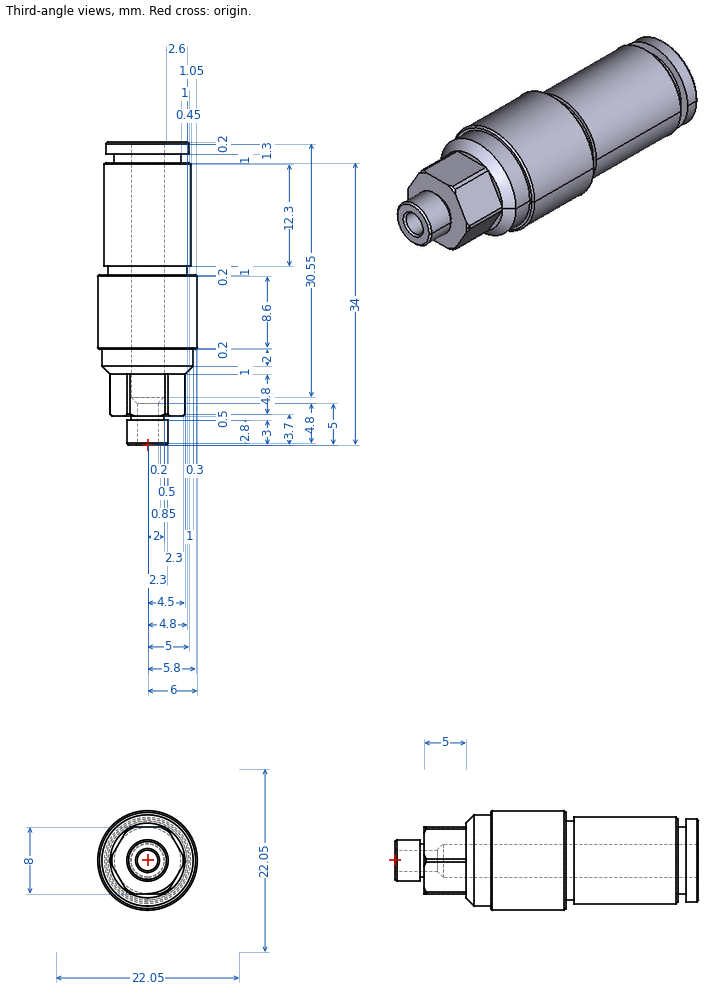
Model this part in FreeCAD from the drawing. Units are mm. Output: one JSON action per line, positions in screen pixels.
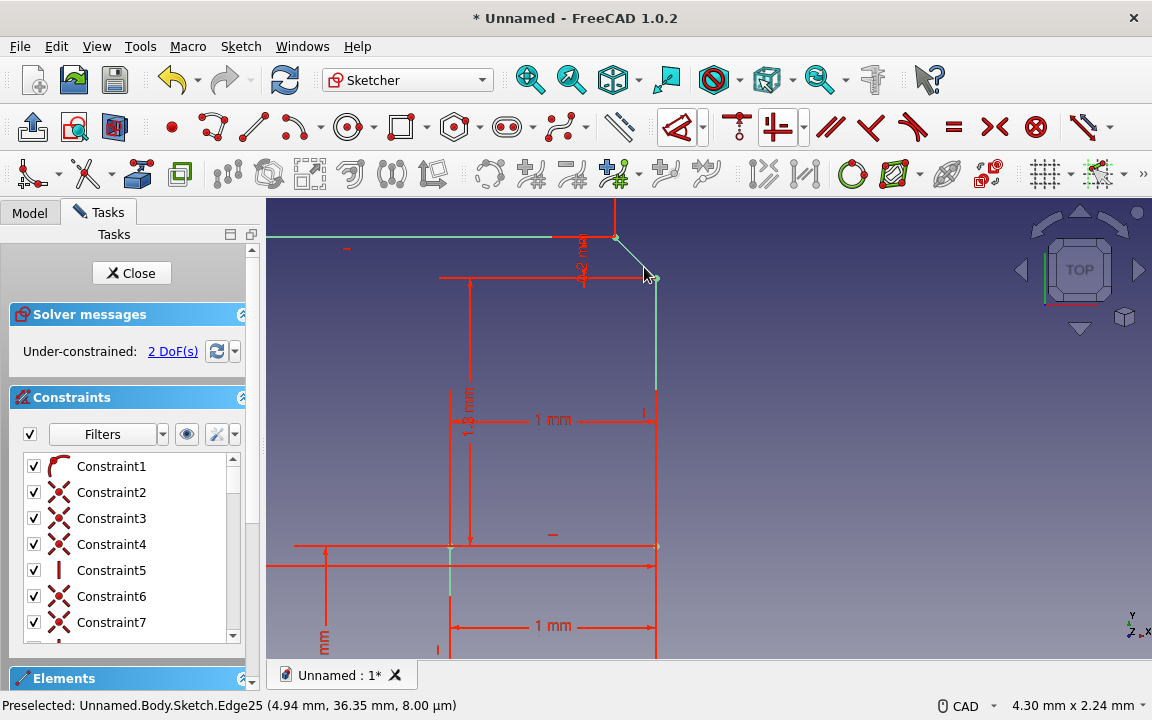
{"action": "scroll", "coordinate": [657, 277], "scroll_direction": "down", "scroll_amount": 16}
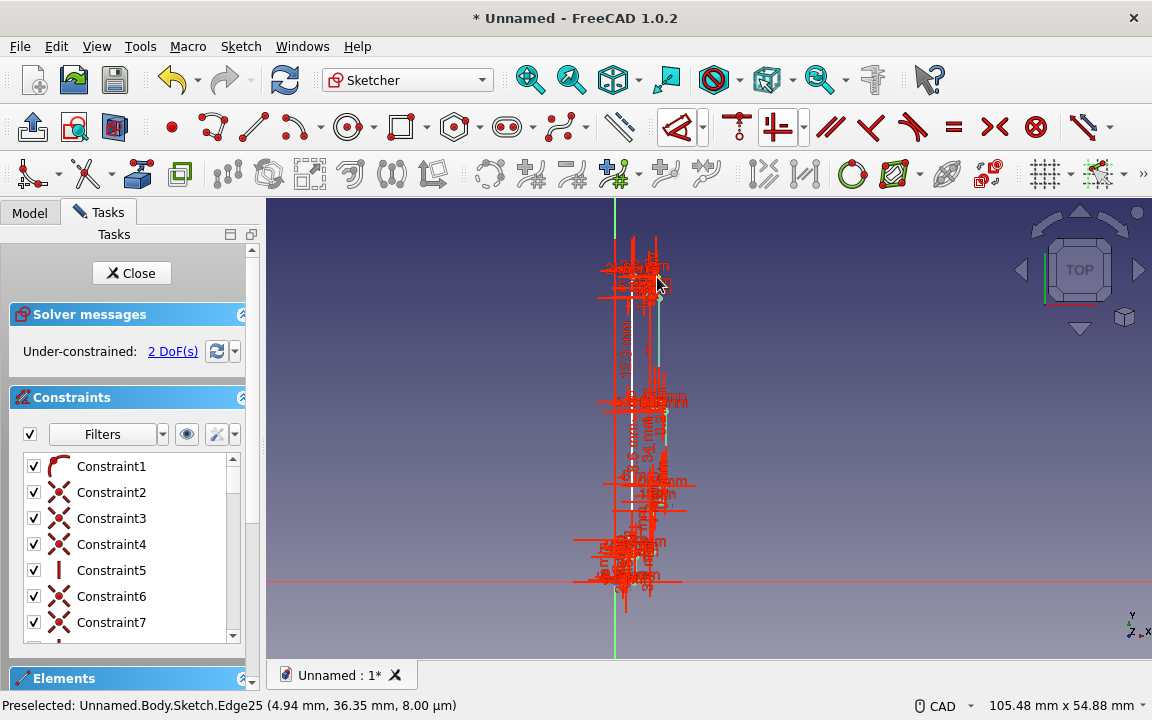
{"action": "scroll", "coordinate": [633, 276], "scroll_direction": "up", "scroll_amount": 16}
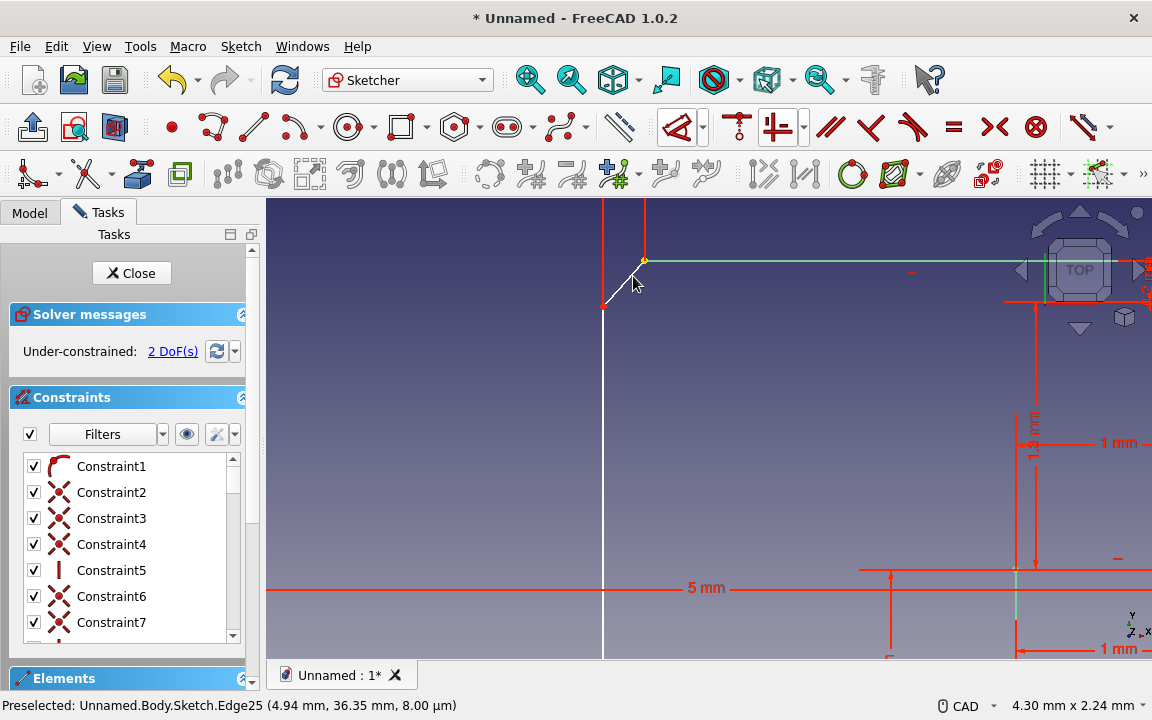
{"action": "left_click", "coordinate": [632, 274]}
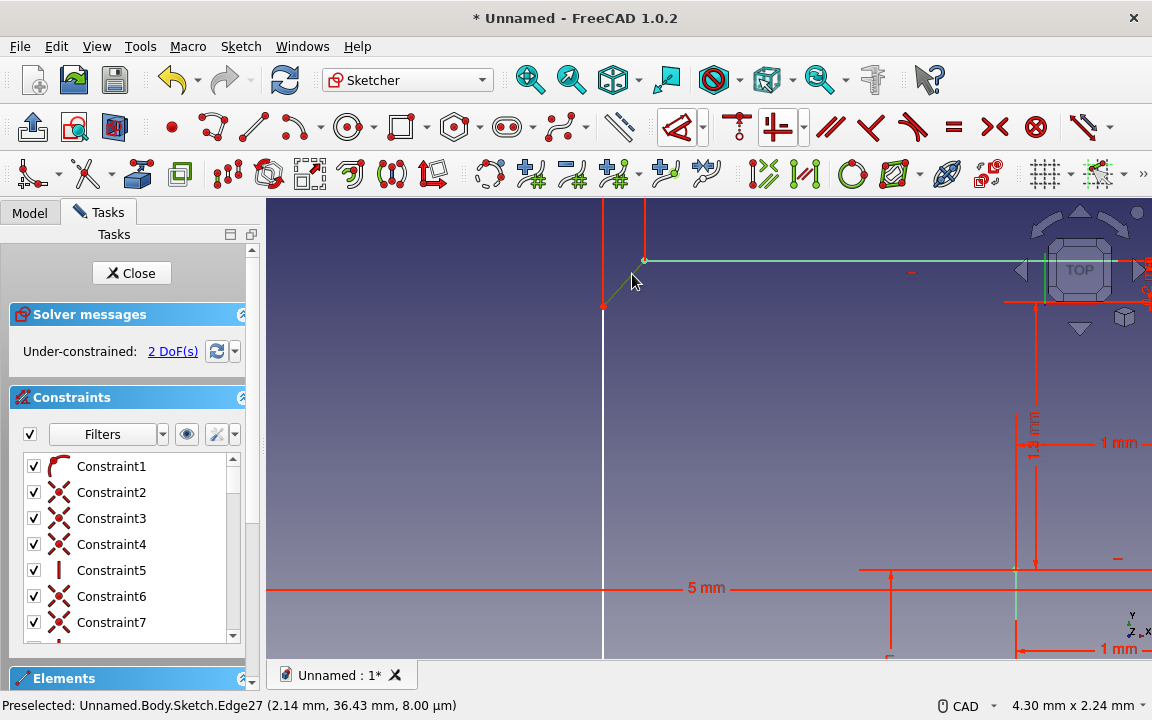
{"action": "left_click", "coordinate": [702, 128]}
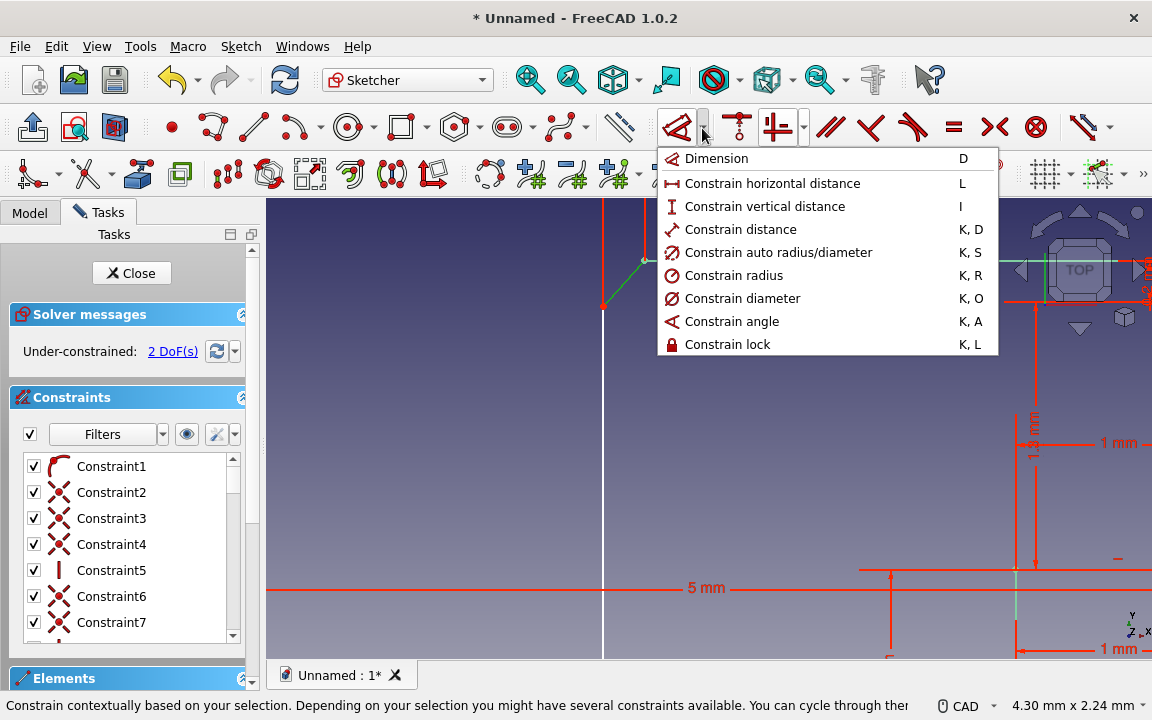
{"action": "left_click", "coordinate": [828, 206]}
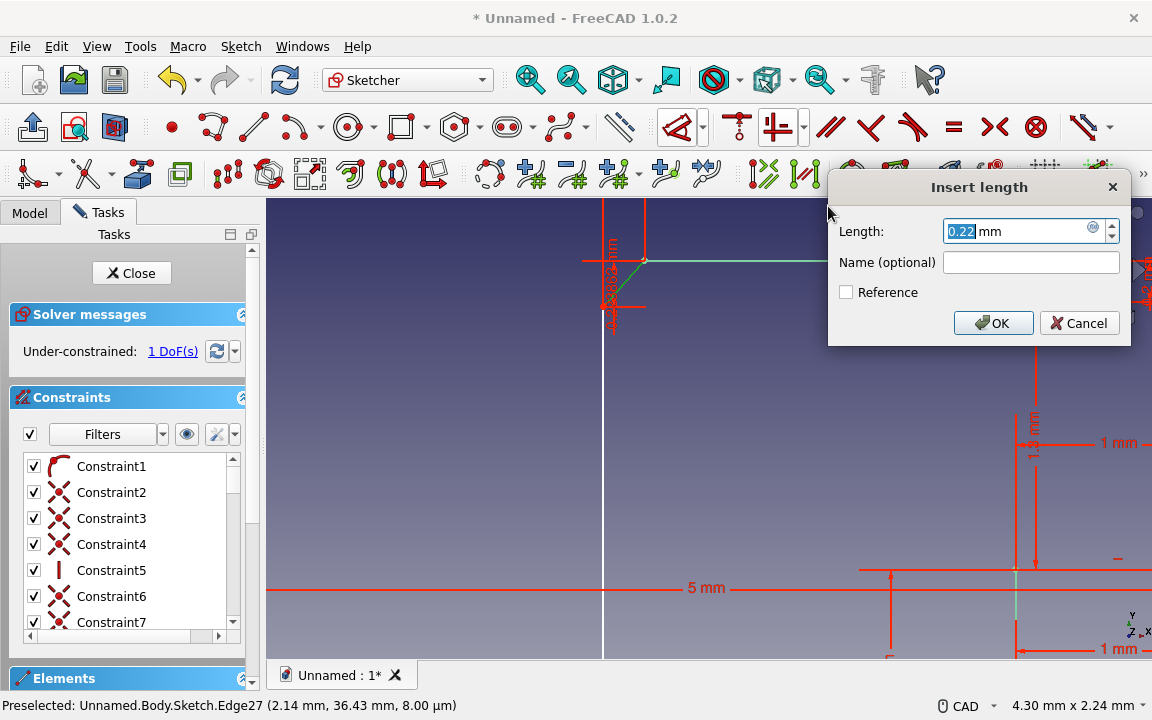
{"action": "type", "text": "0.2"}
{"action": "key", "text": "Return"}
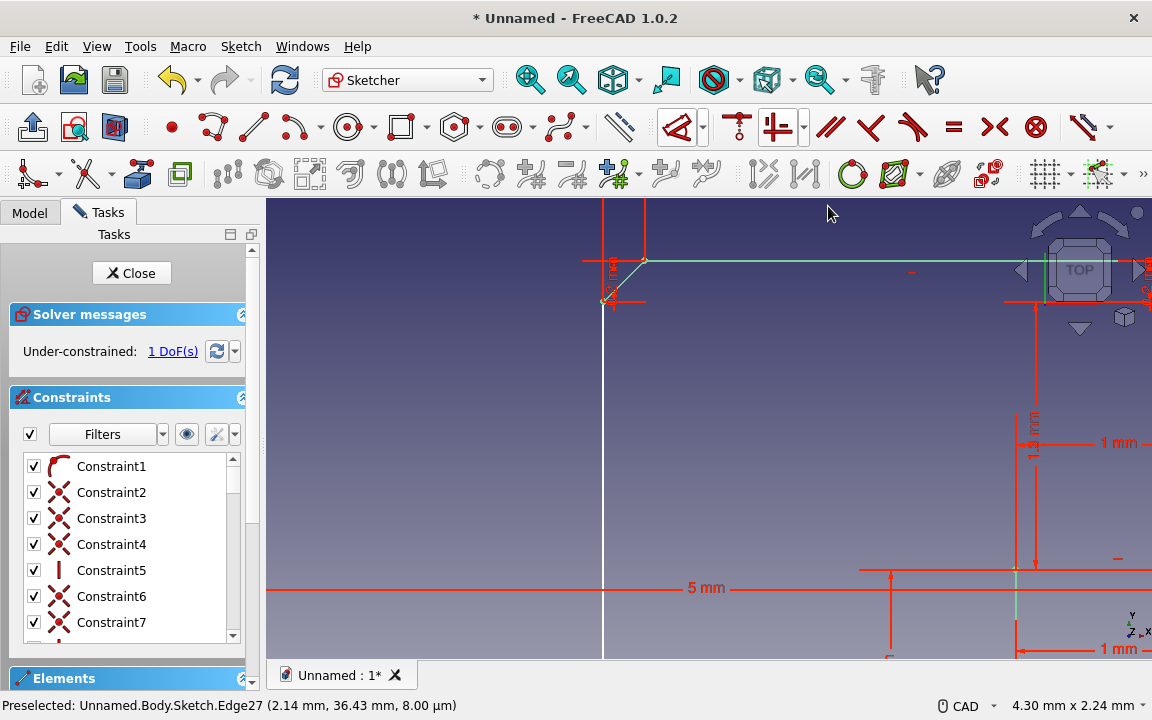
{"action": "scroll", "coordinate": [633, 276], "scroll_direction": "down", "scroll_amount": 16}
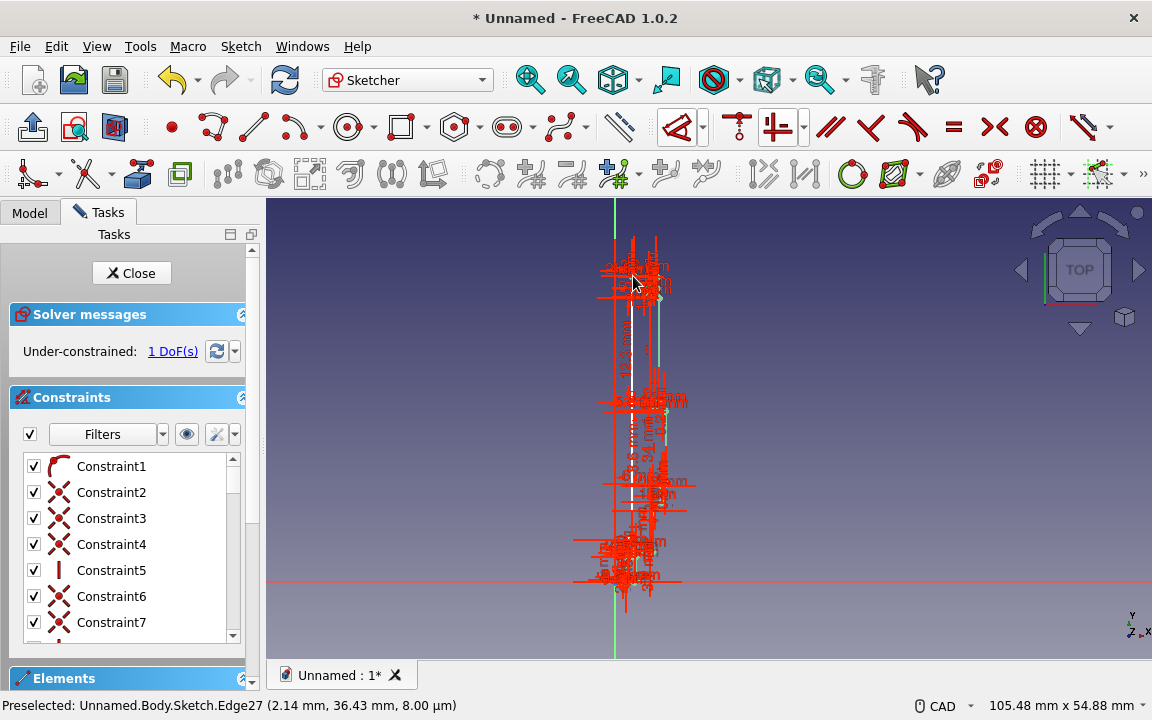
{"action": "left_click", "coordinate": [632, 380]}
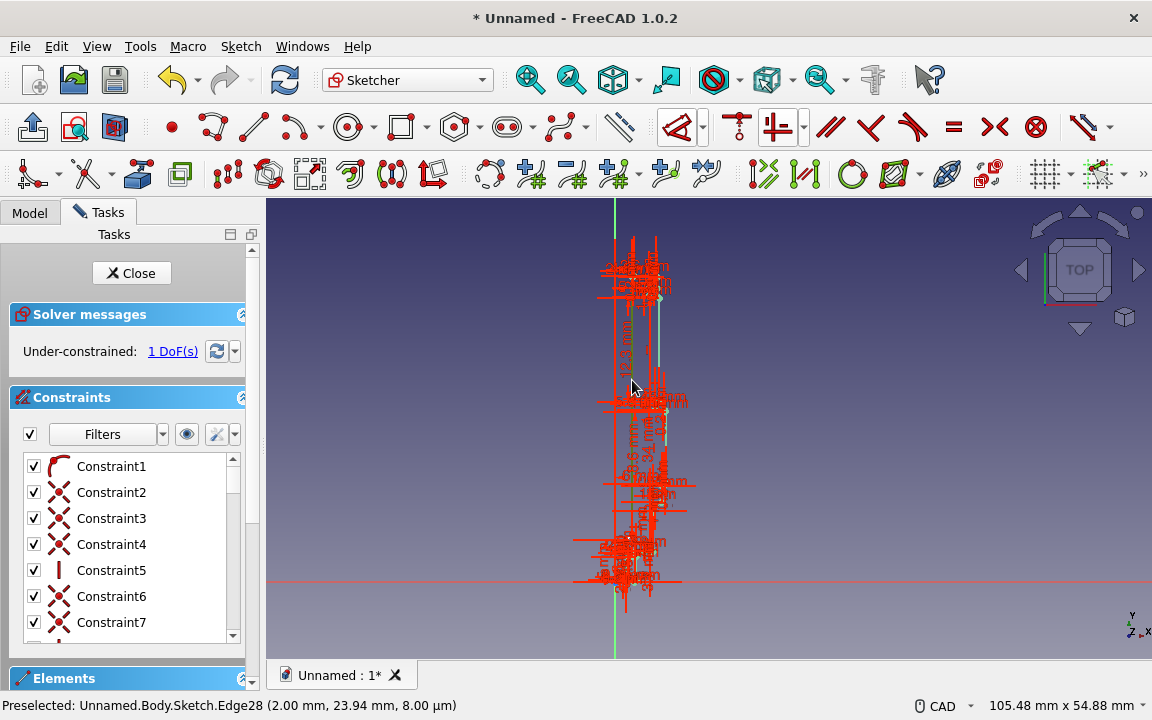
{"action": "key", "text": "i"}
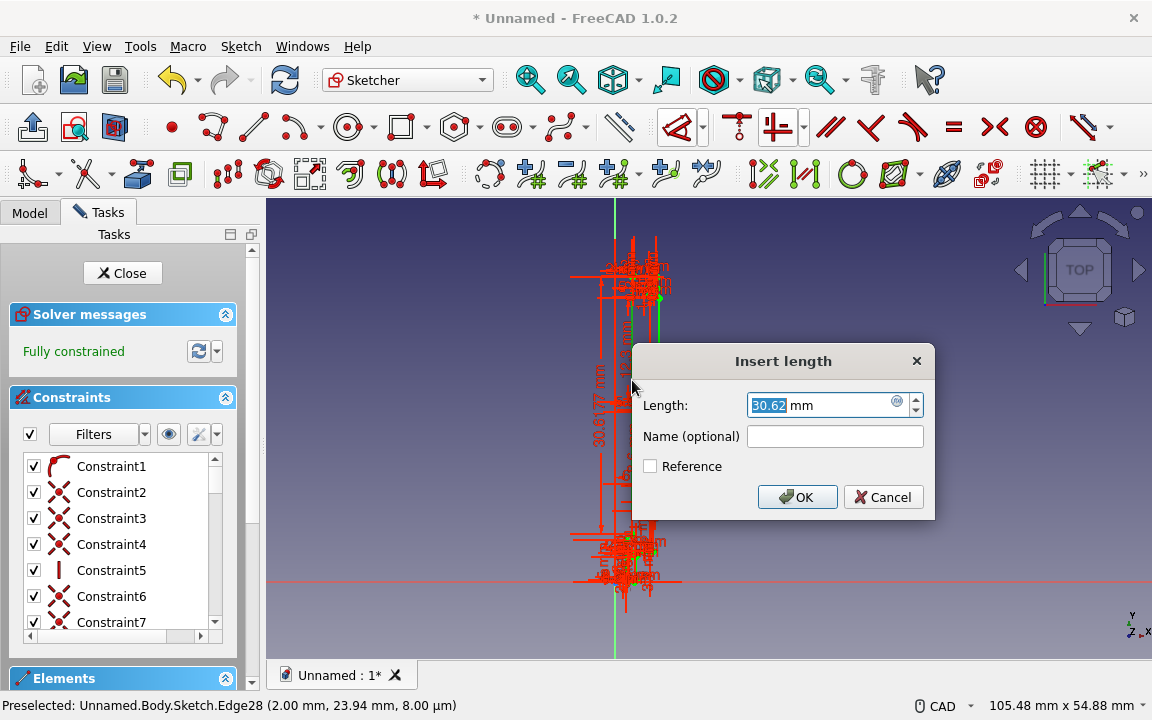
{"action": "type", "text": "30.55"}
{"action": "key", "text": "Return"}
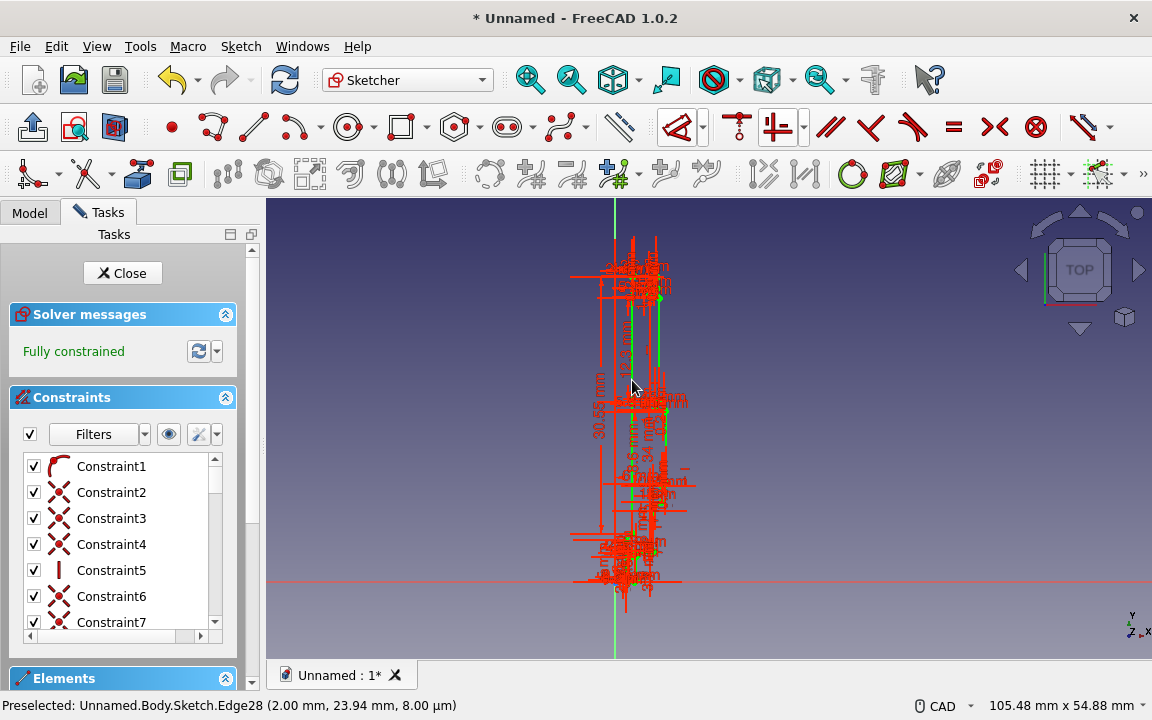
{"action": "left_click", "coordinate": [123, 273]}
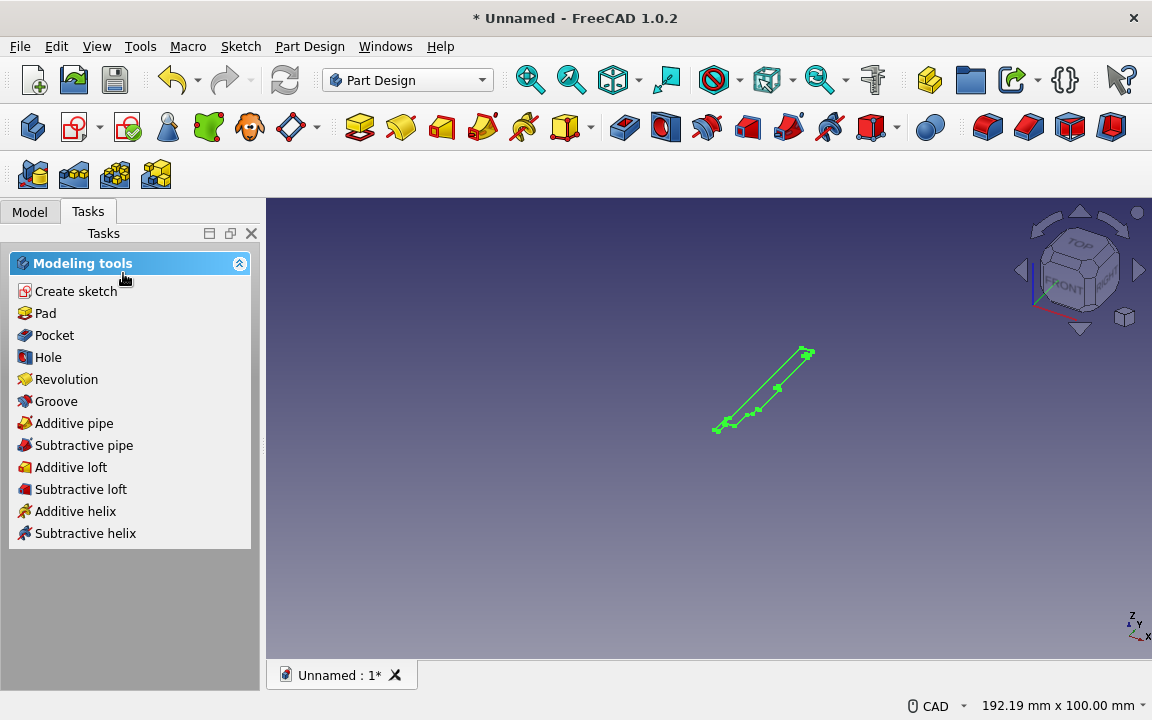
{"action": "left_click", "coordinate": [401, 128]}